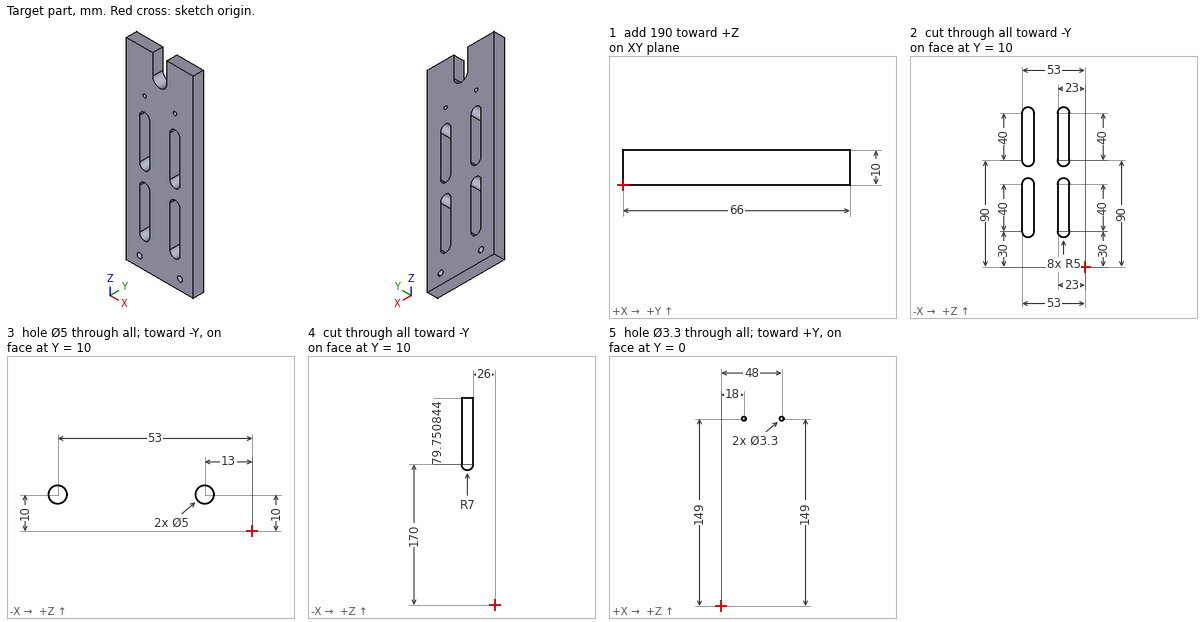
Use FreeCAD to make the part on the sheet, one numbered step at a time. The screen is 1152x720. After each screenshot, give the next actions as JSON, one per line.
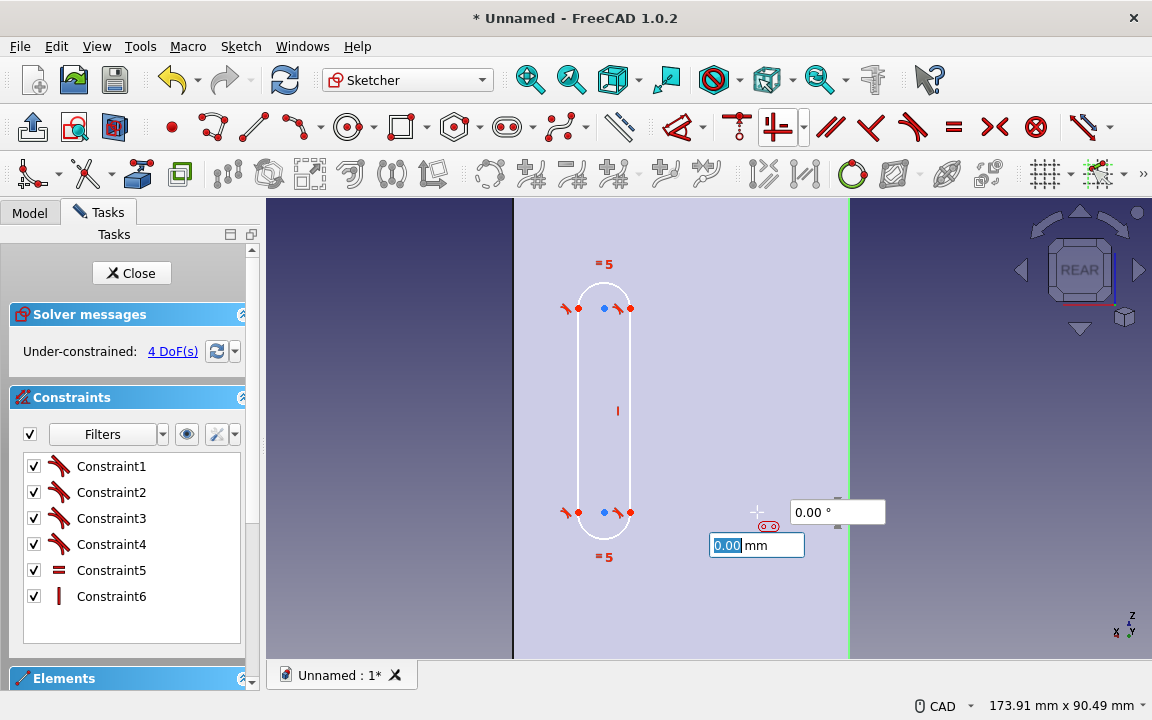
{"action": "left_click", "coordinate": [757, 308]}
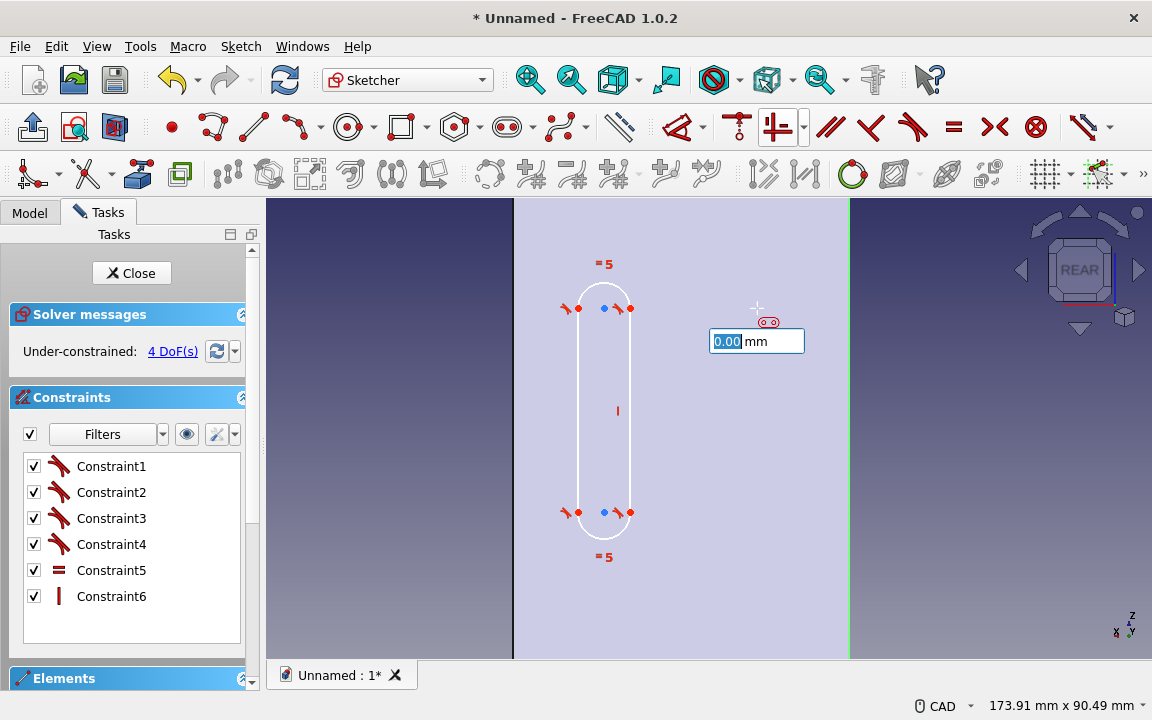
{"action": "left_click", "coordinate": [783, 410]}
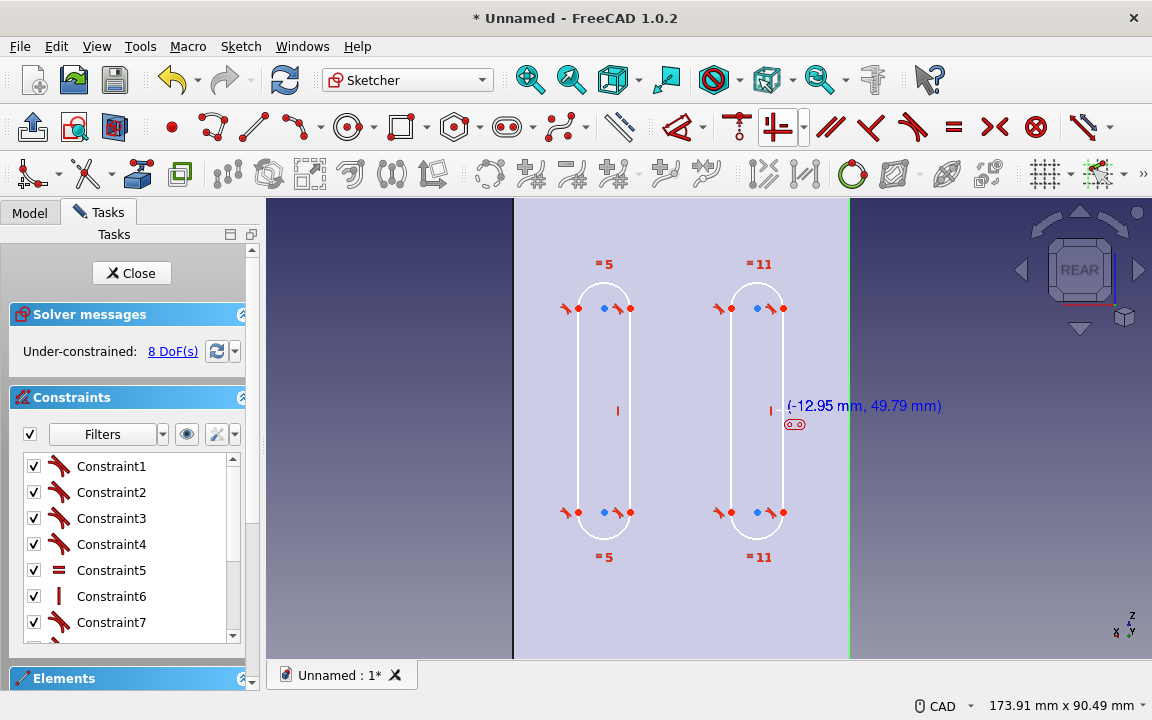
{"action": "scroll", "coordinate": [581, 516], "scroll_direction": "down", "scroll_amount": 4}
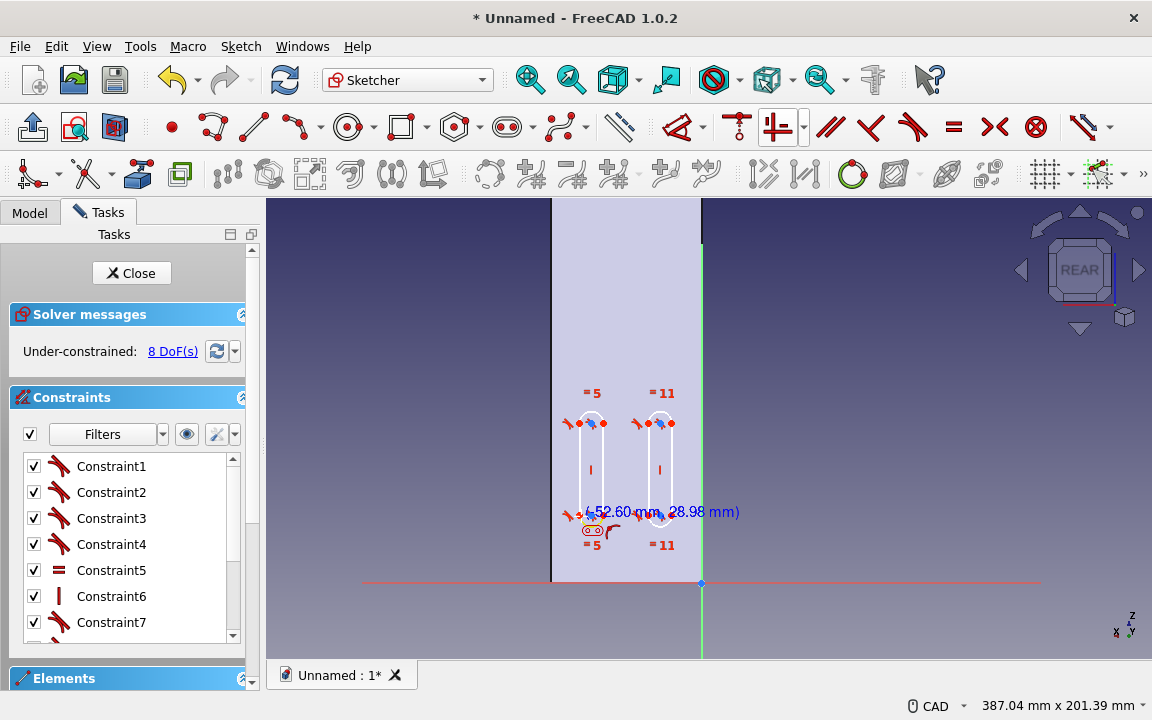
{"action": "scroll", "coordinate": [592, 377], "scroll_direction": "up", "scroll_amount": 4}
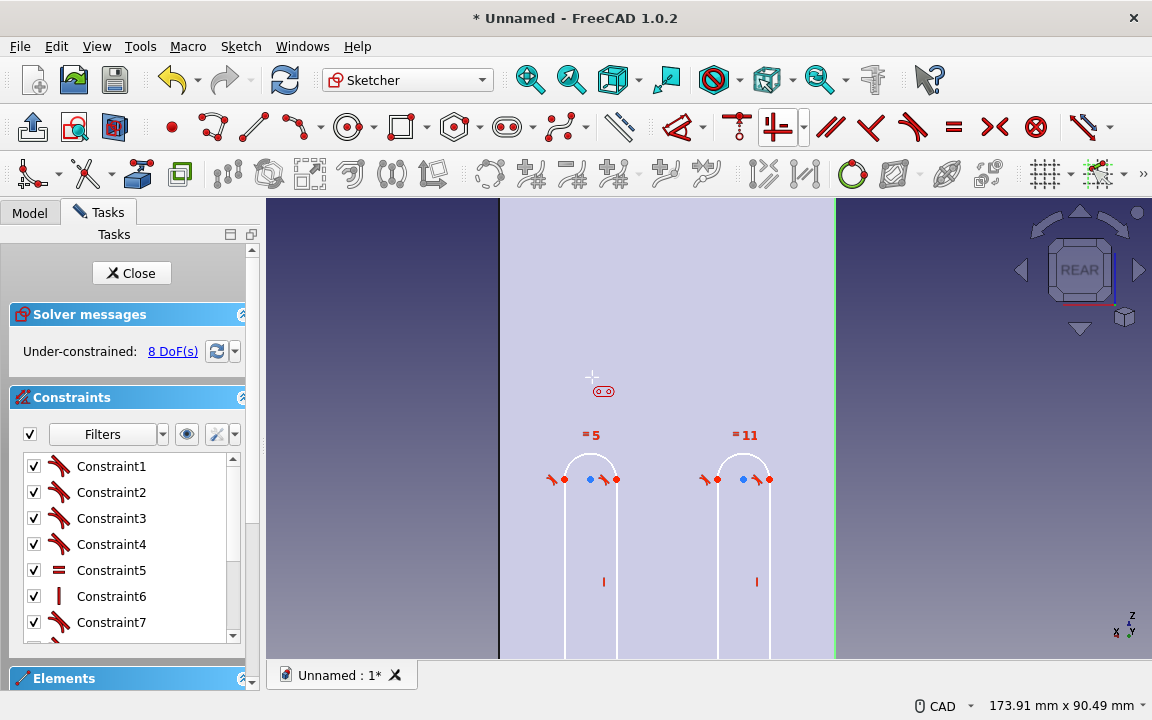
{"action": "left_click", "coordinate": [591, 377]}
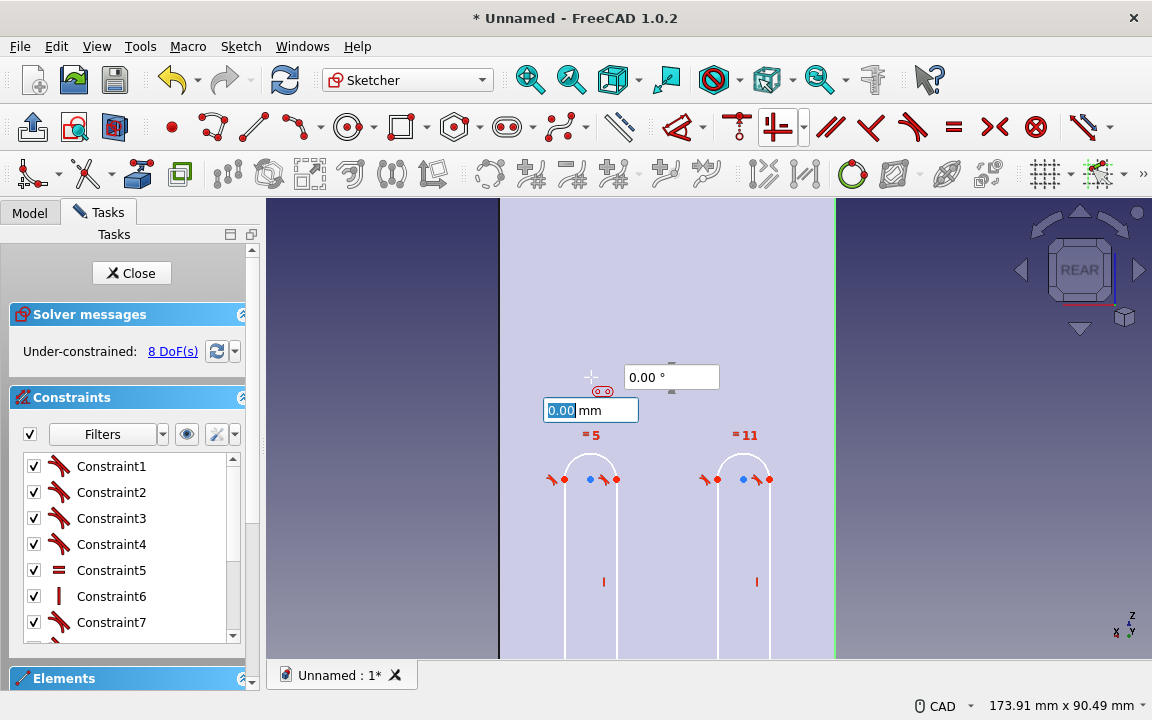
{"action": "scroll", "coordinate": [592, 377], "scroll_direction": "down", "scroll_amount": 4}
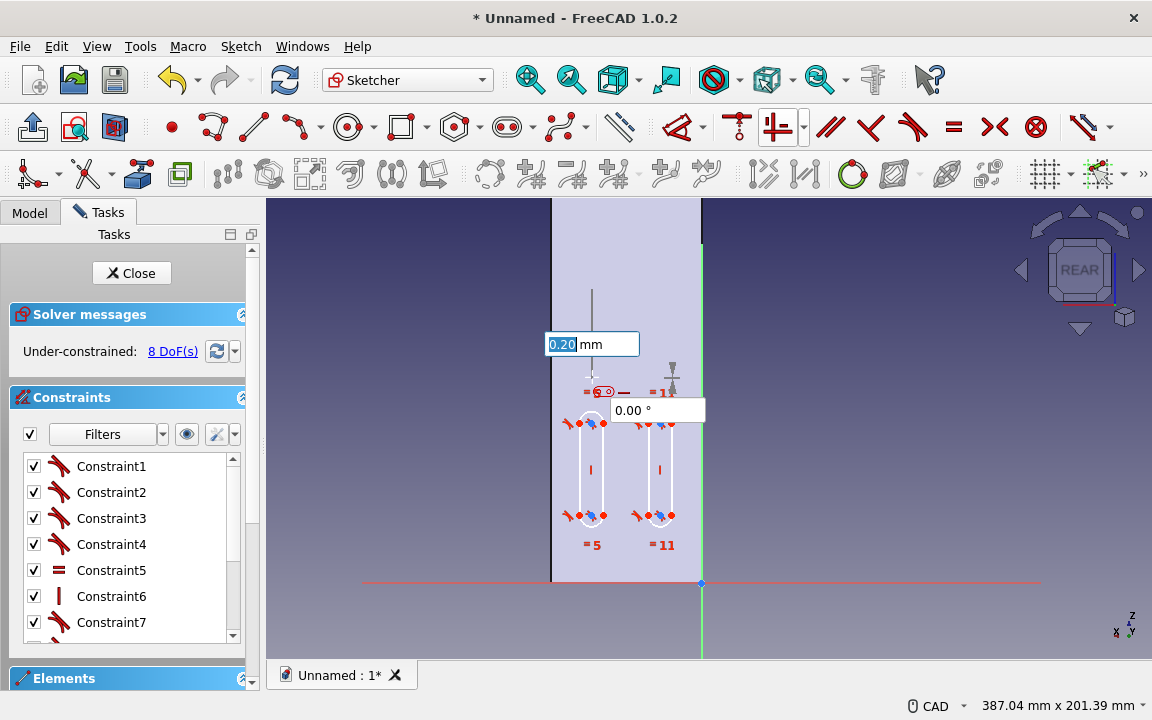
{"action": "left_click", "coordinate": [592, 286]}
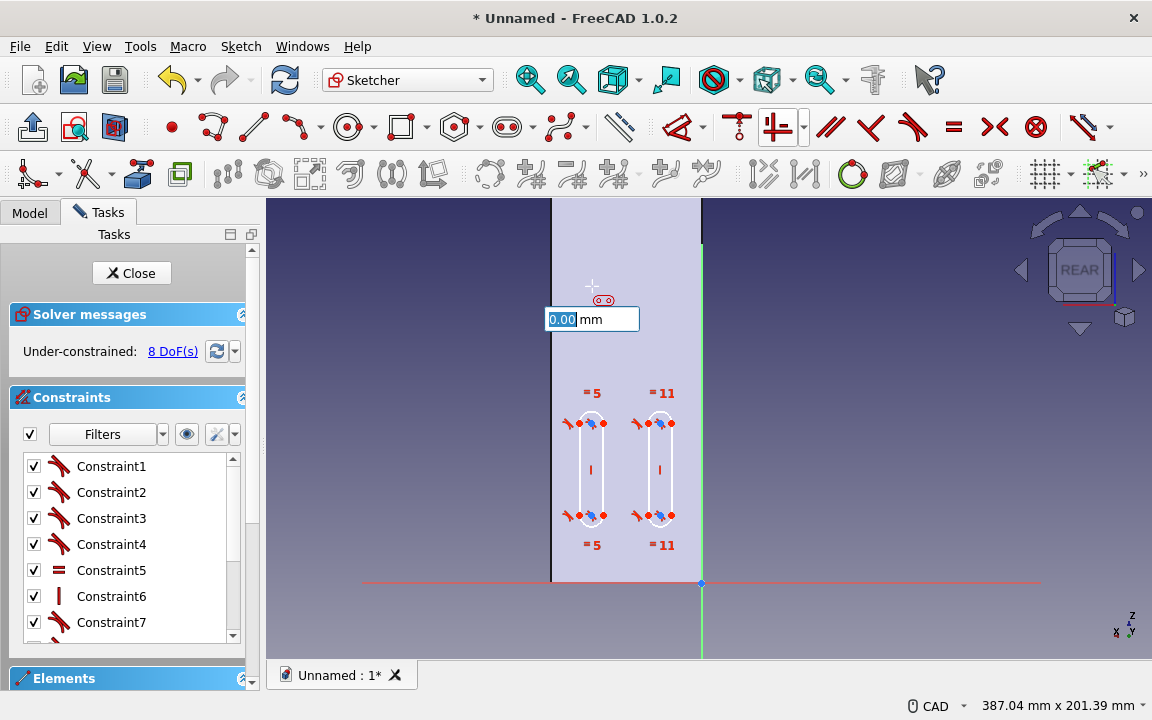
{"action": "scroll", "coordinate": [603, 331], "scroll_direction": "up", "scroll_amount": 2}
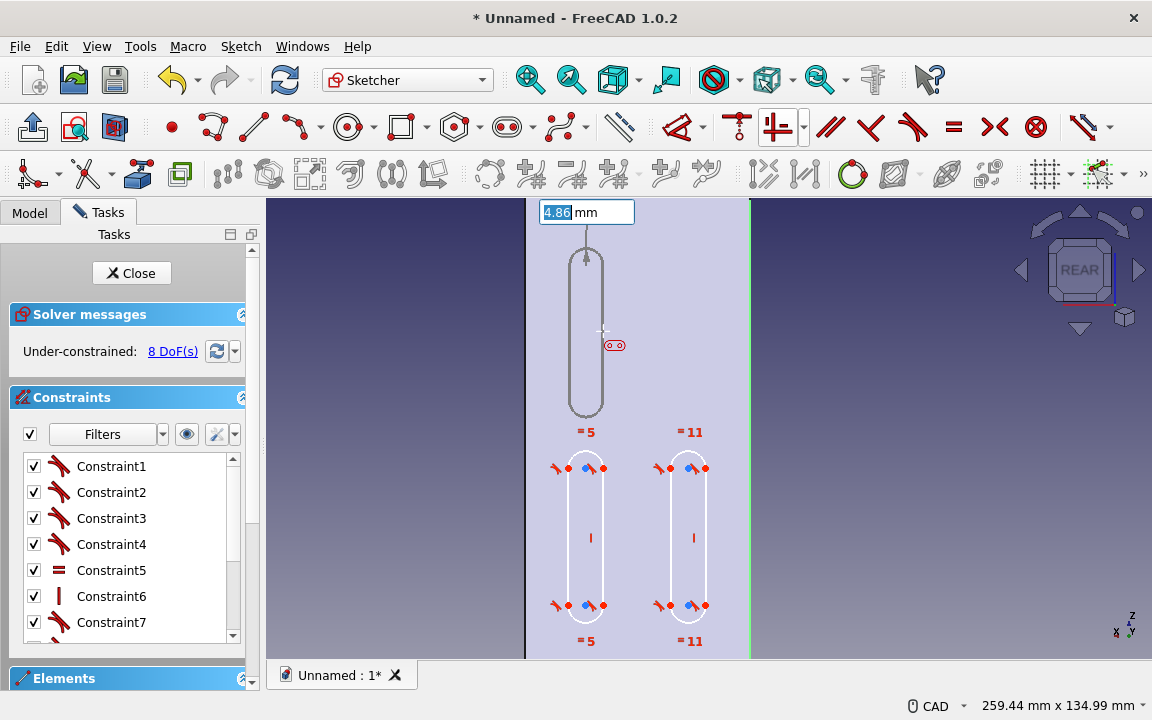
{"action": "left_click", "coordinate": [603, 331]}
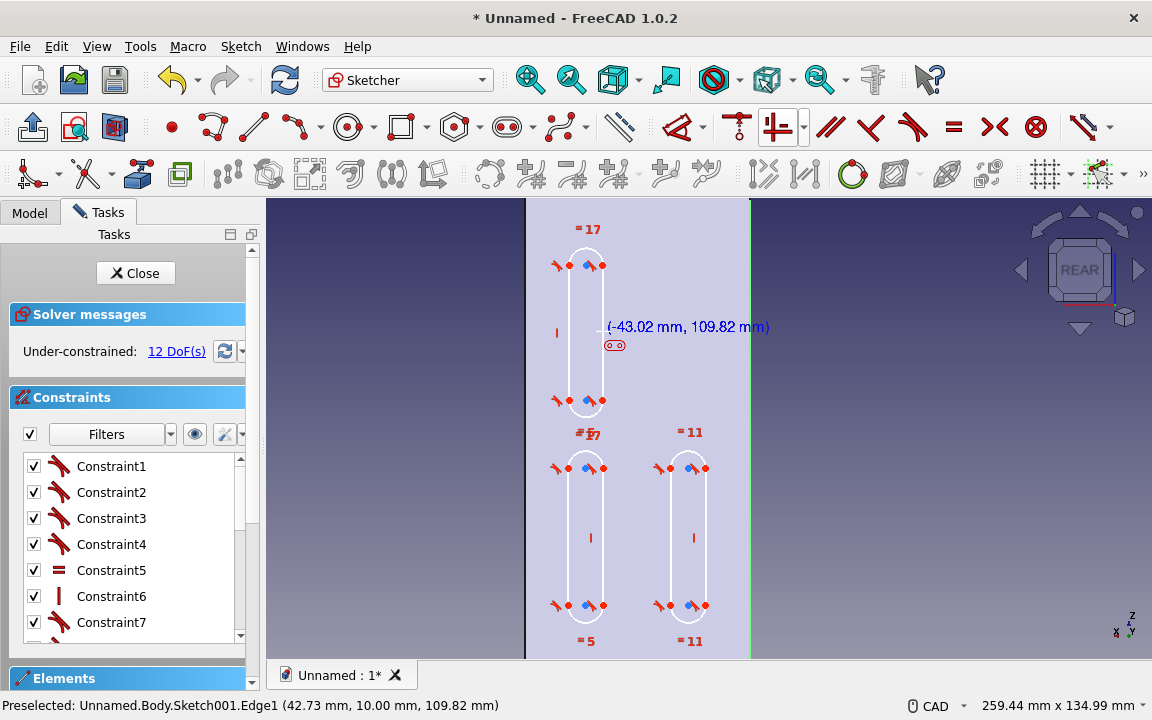
{"action": "scroll", "coordinate": [688, 400], "scroll_direction": "up", "scroll_amount": 2}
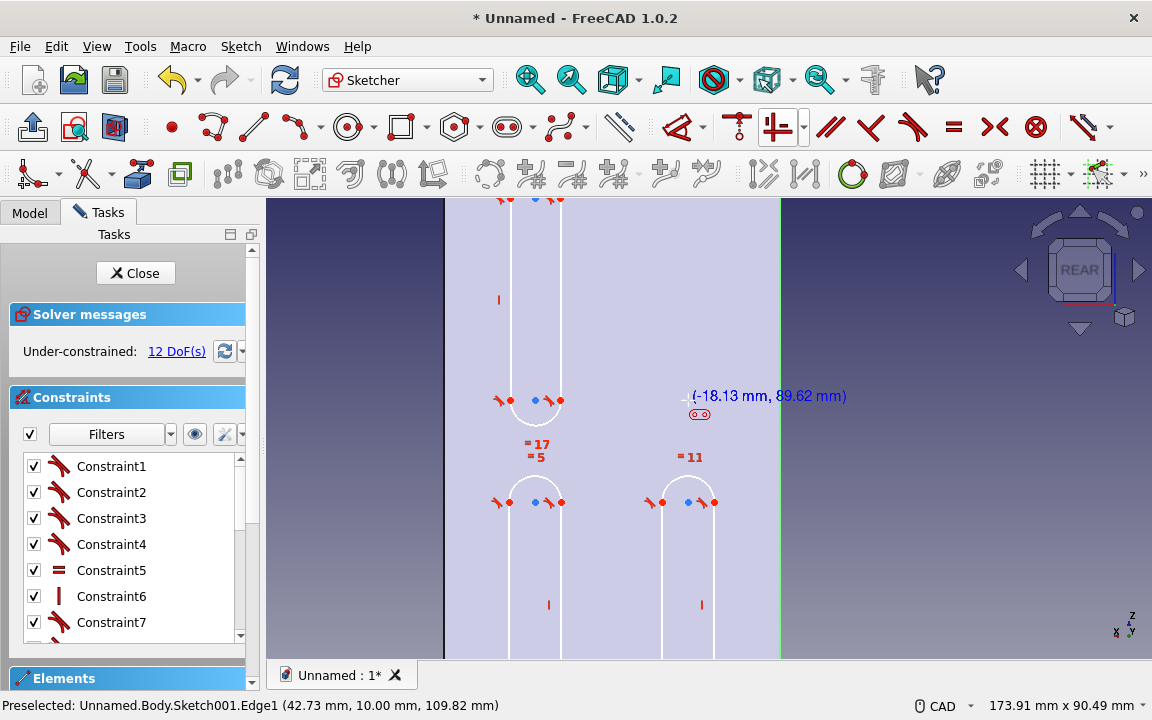
{"action": "left_click", "coordinate": [688, 399]}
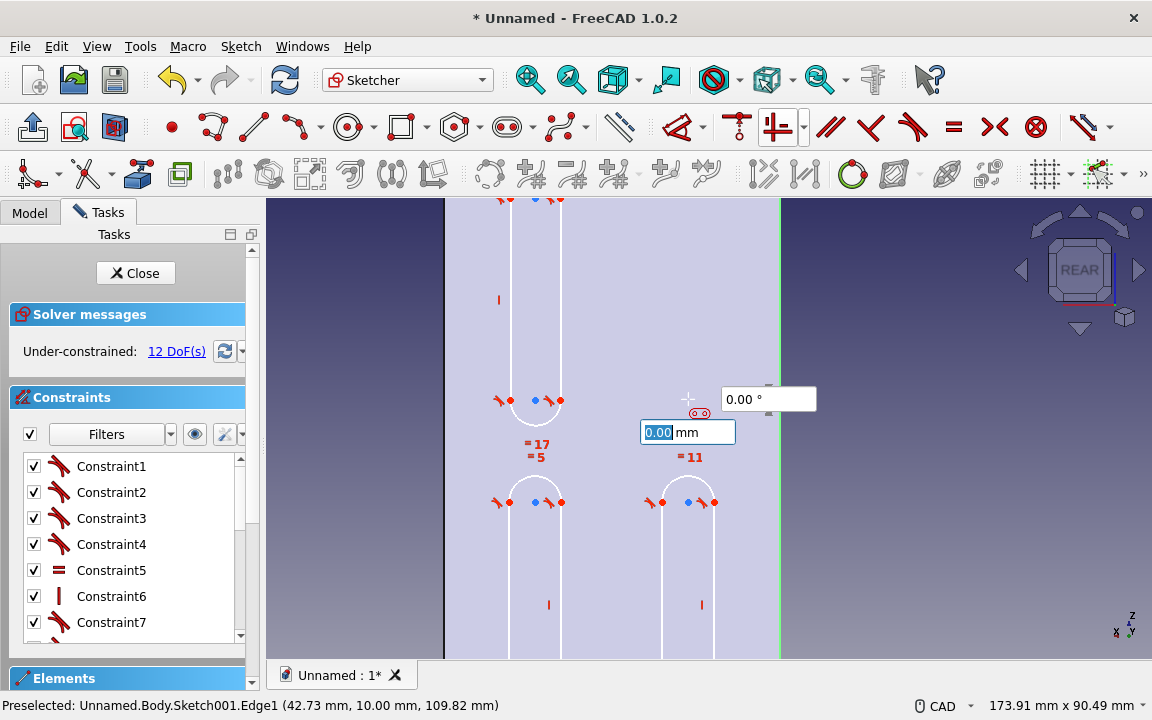
{"action": "scroll", "coordinate": [637, 359], "scroll_direction": "down", "scroll_amount": 4}